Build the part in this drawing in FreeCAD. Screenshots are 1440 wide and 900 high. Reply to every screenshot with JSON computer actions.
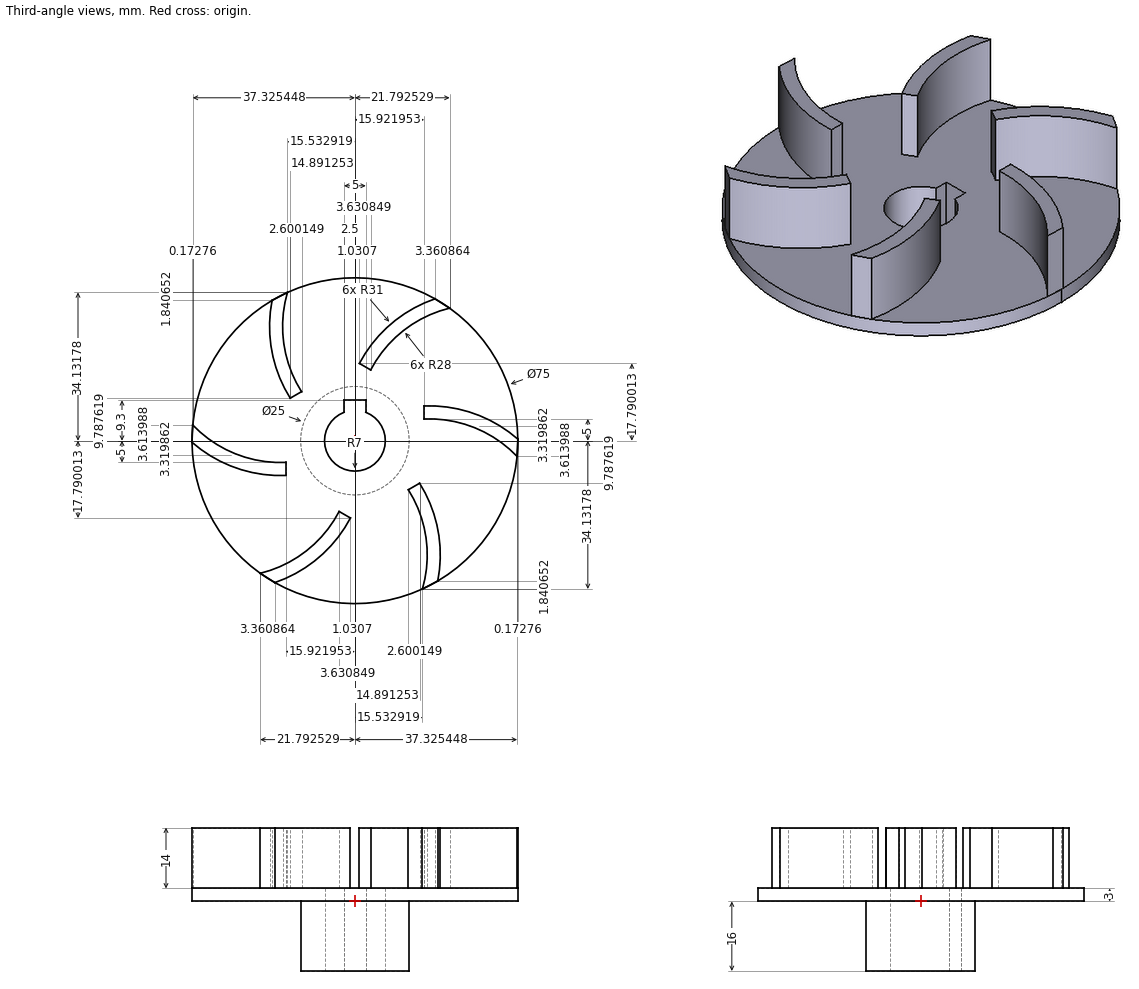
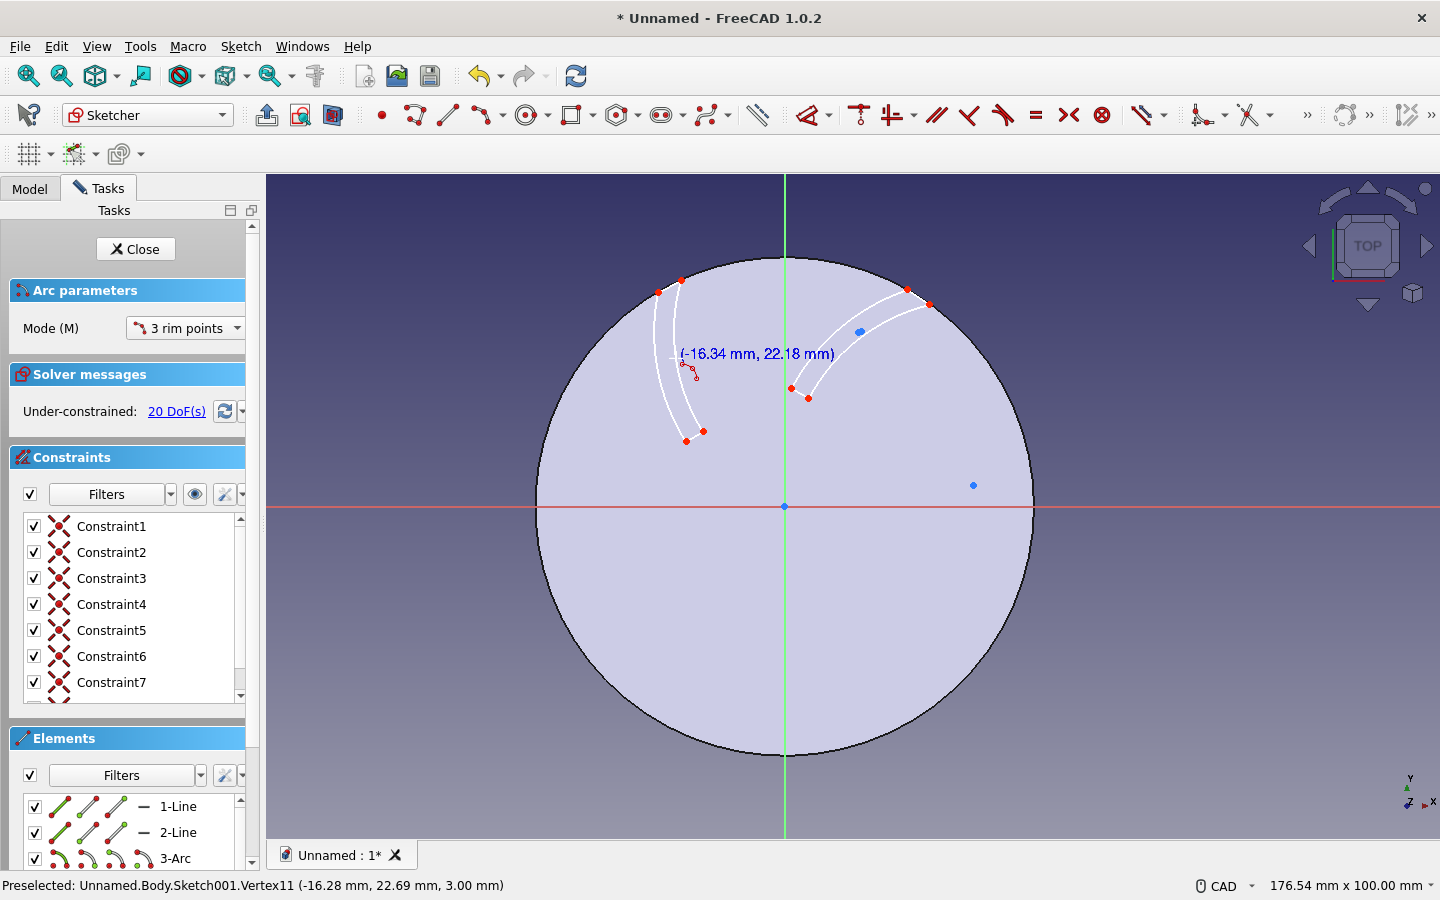
{"action": "key", "text": "g l"}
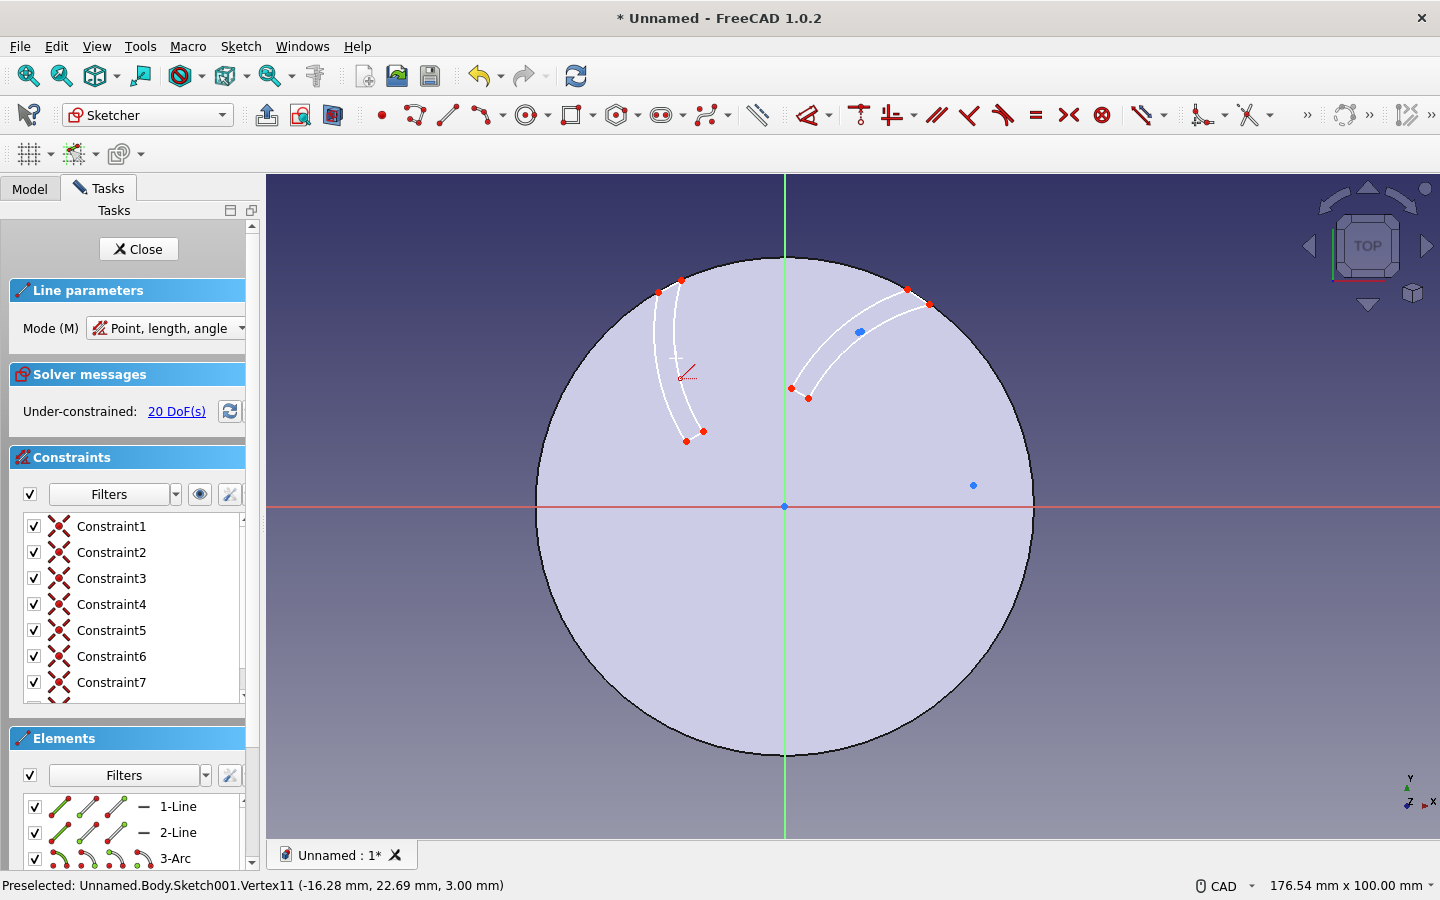
{"action": "left_click", "coordinate": [536, 482]}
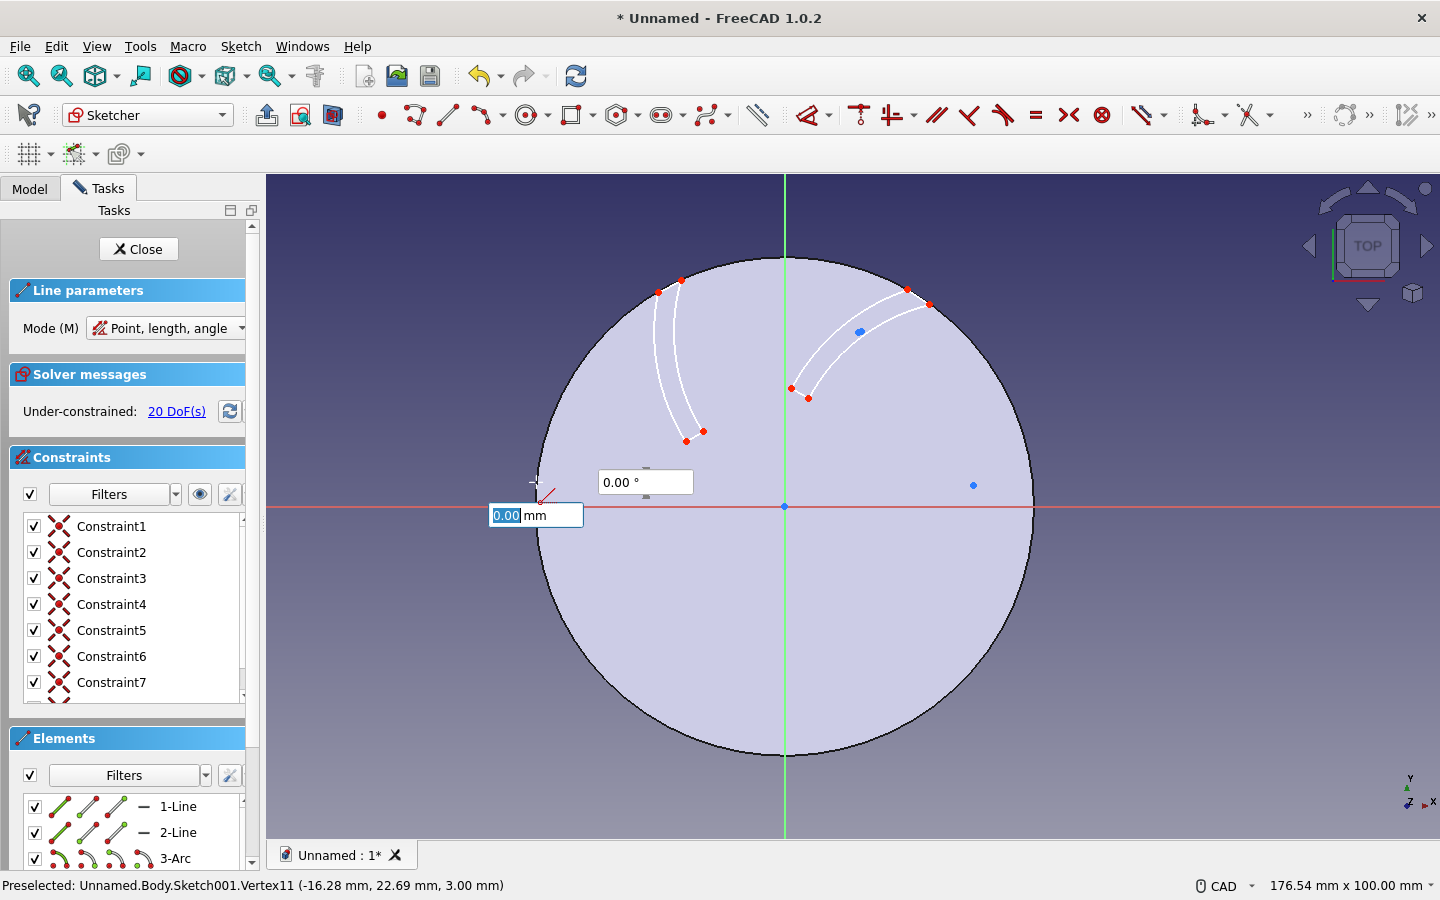
{"action": "scroll", "coordinate": [535, 509], "scroll_direction": "up", "scroll_amount": 10}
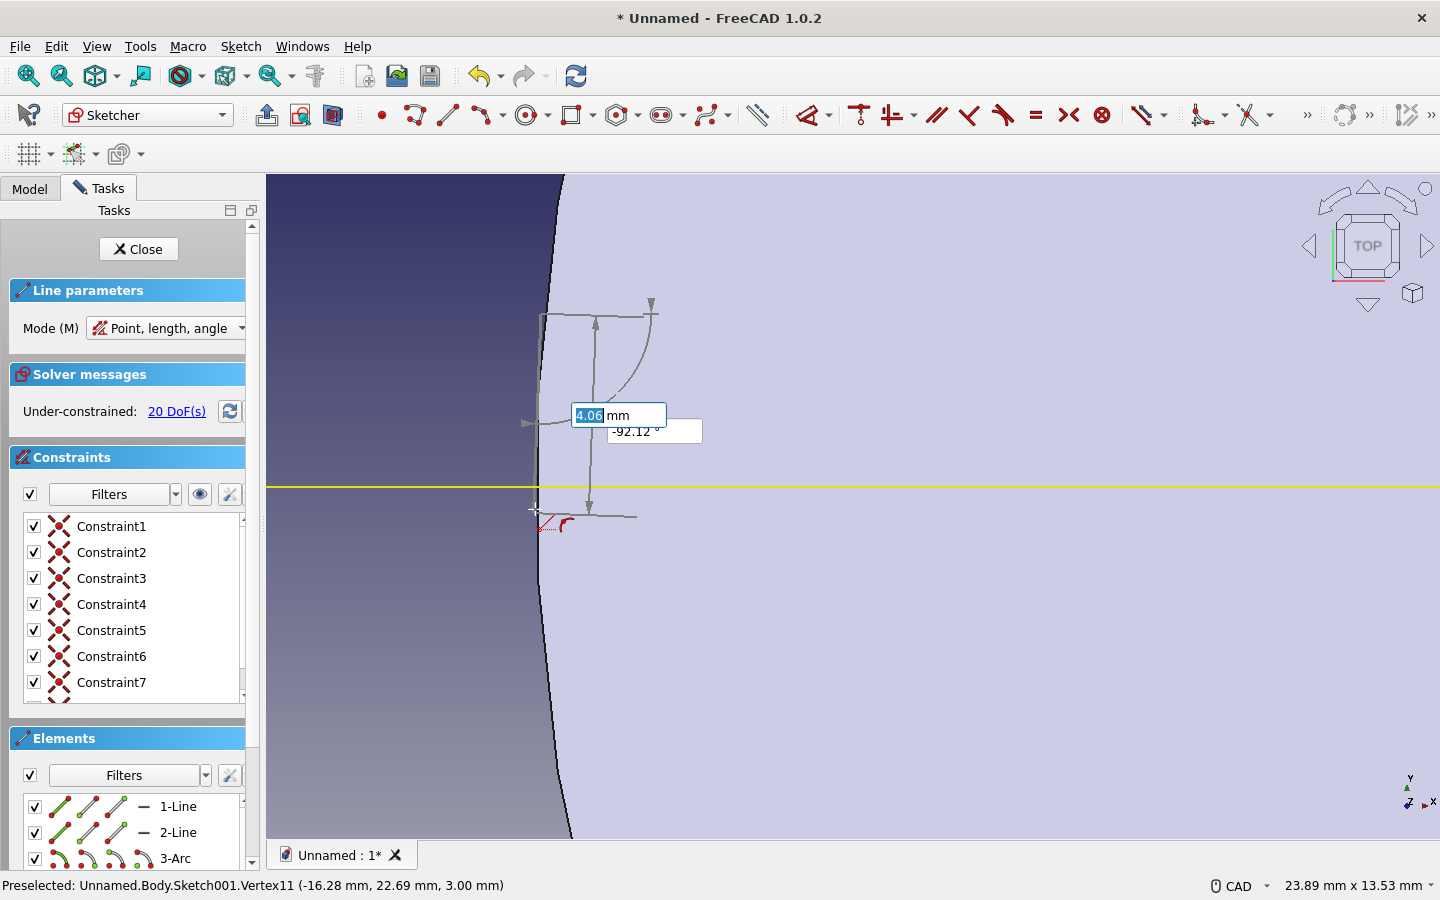
{"action": "left_click", "coordinate": [531, 505]}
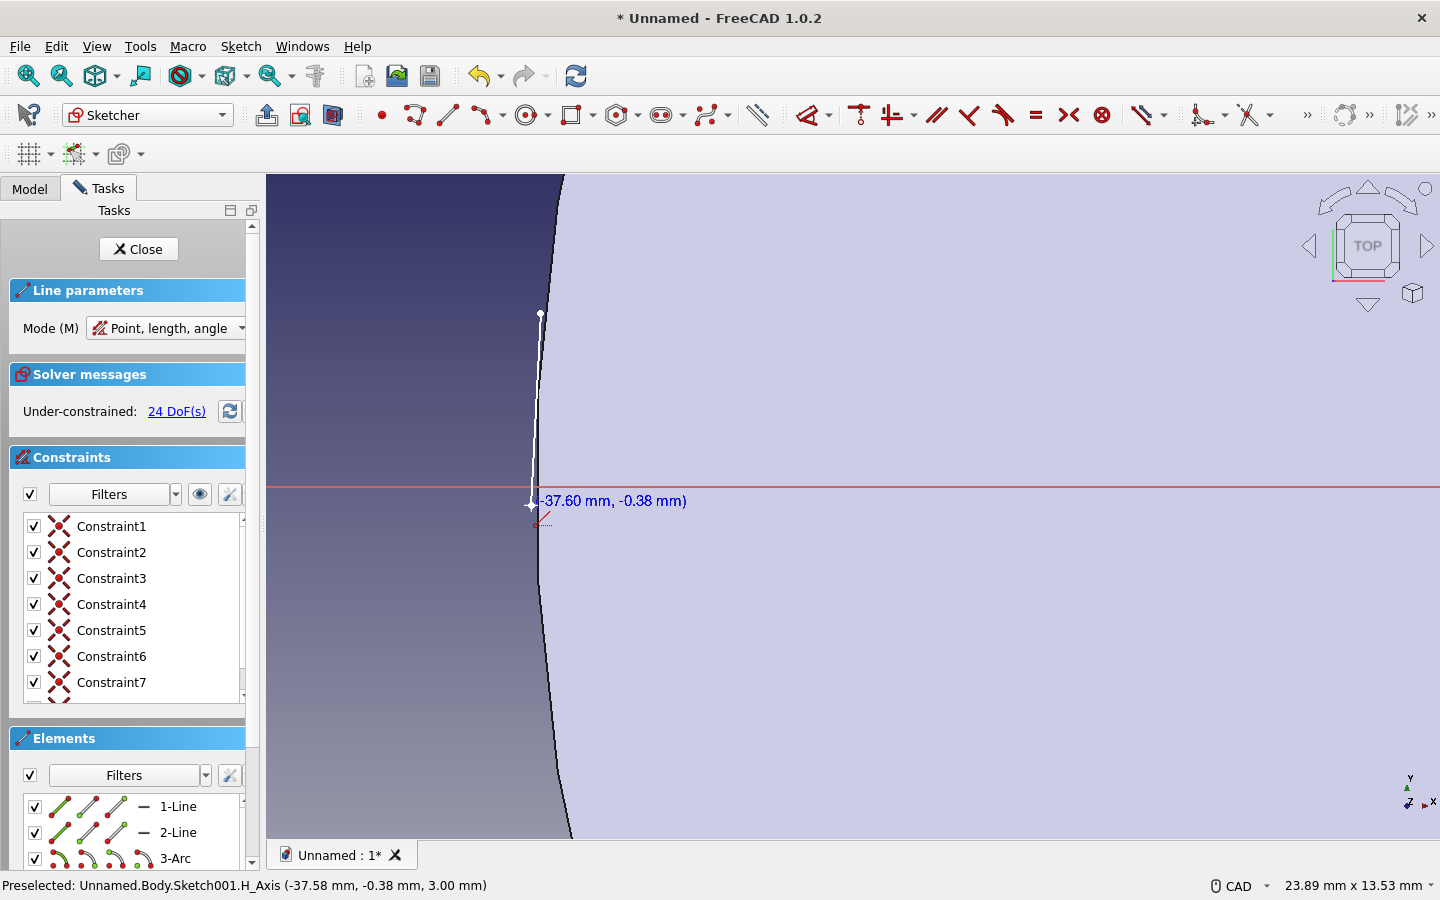
{"action": "scroll", "coordinate": [535, 510], "scroll_direction": "down", "scroll_amount": 10}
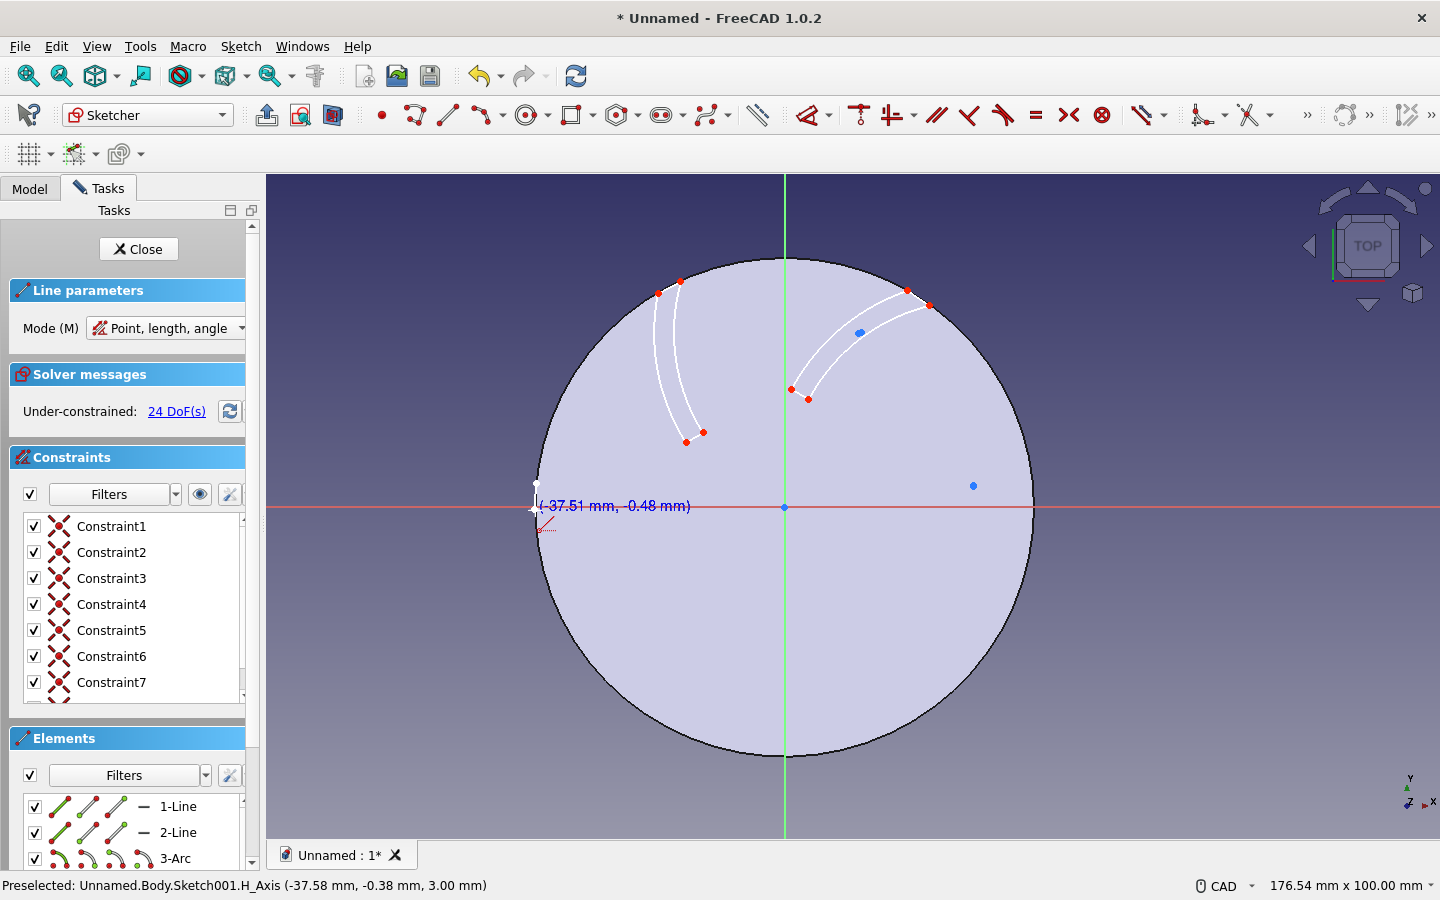
{"action": "left_click", "coordinate": [679, 561]}
{"action": "left_click", "coordinate": [679, 541]}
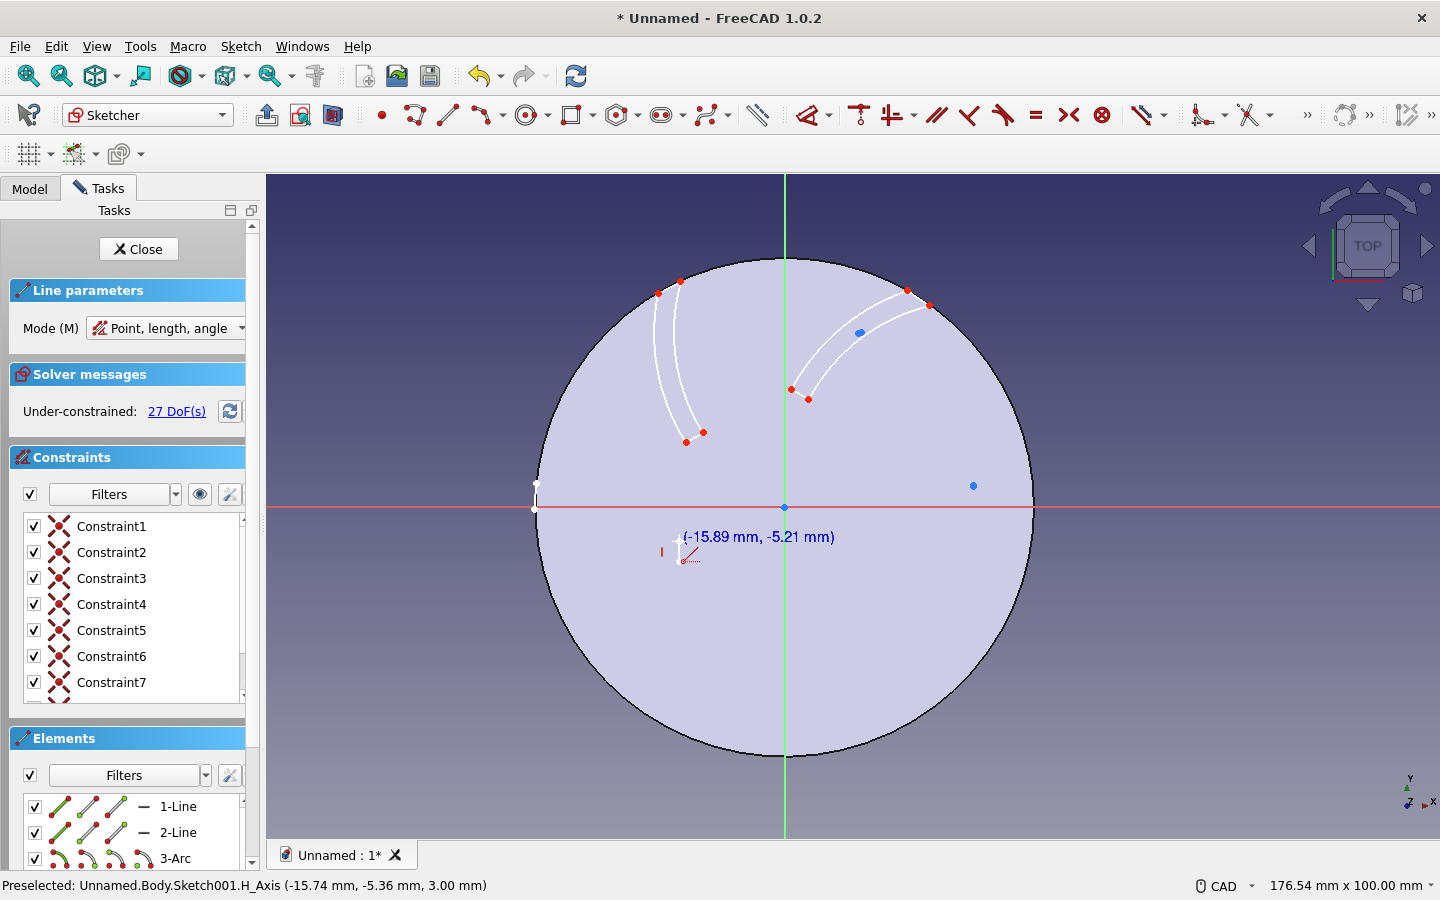
{"action": "key", "text": "g 3 a"}